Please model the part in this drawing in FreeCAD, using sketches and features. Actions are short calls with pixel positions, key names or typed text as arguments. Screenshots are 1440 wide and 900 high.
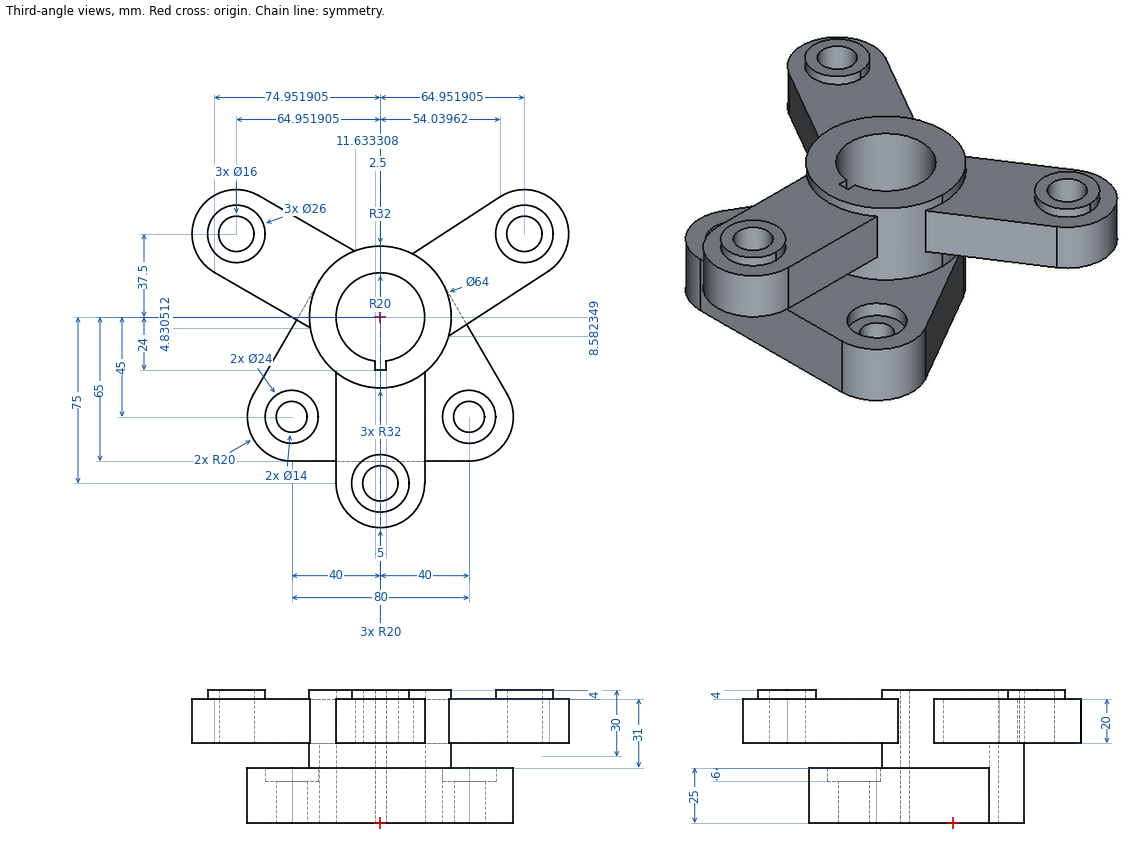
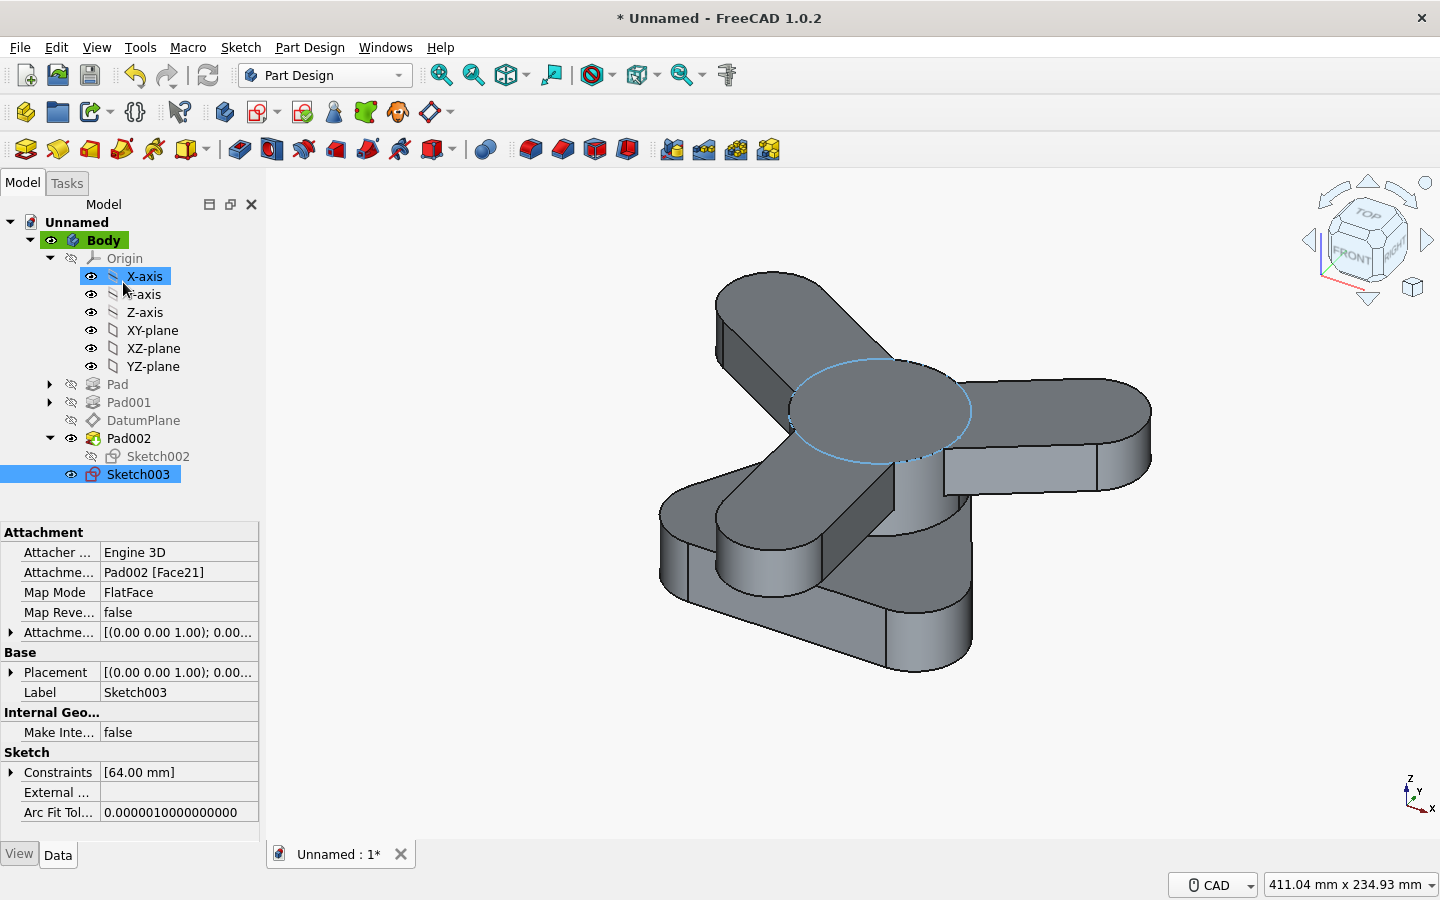
click(26, 150)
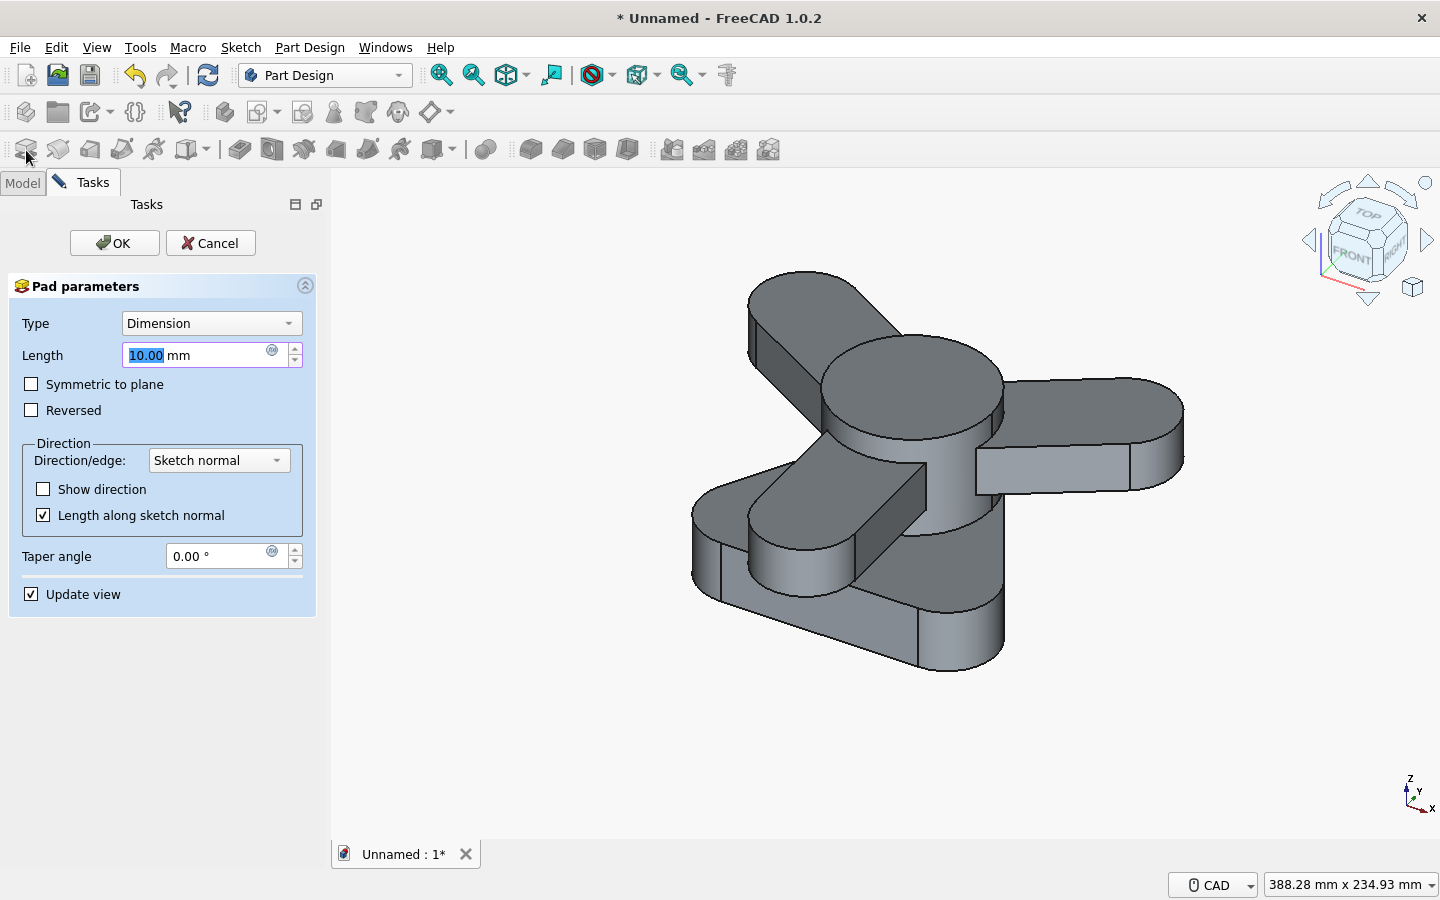
text(4)
key(Tab)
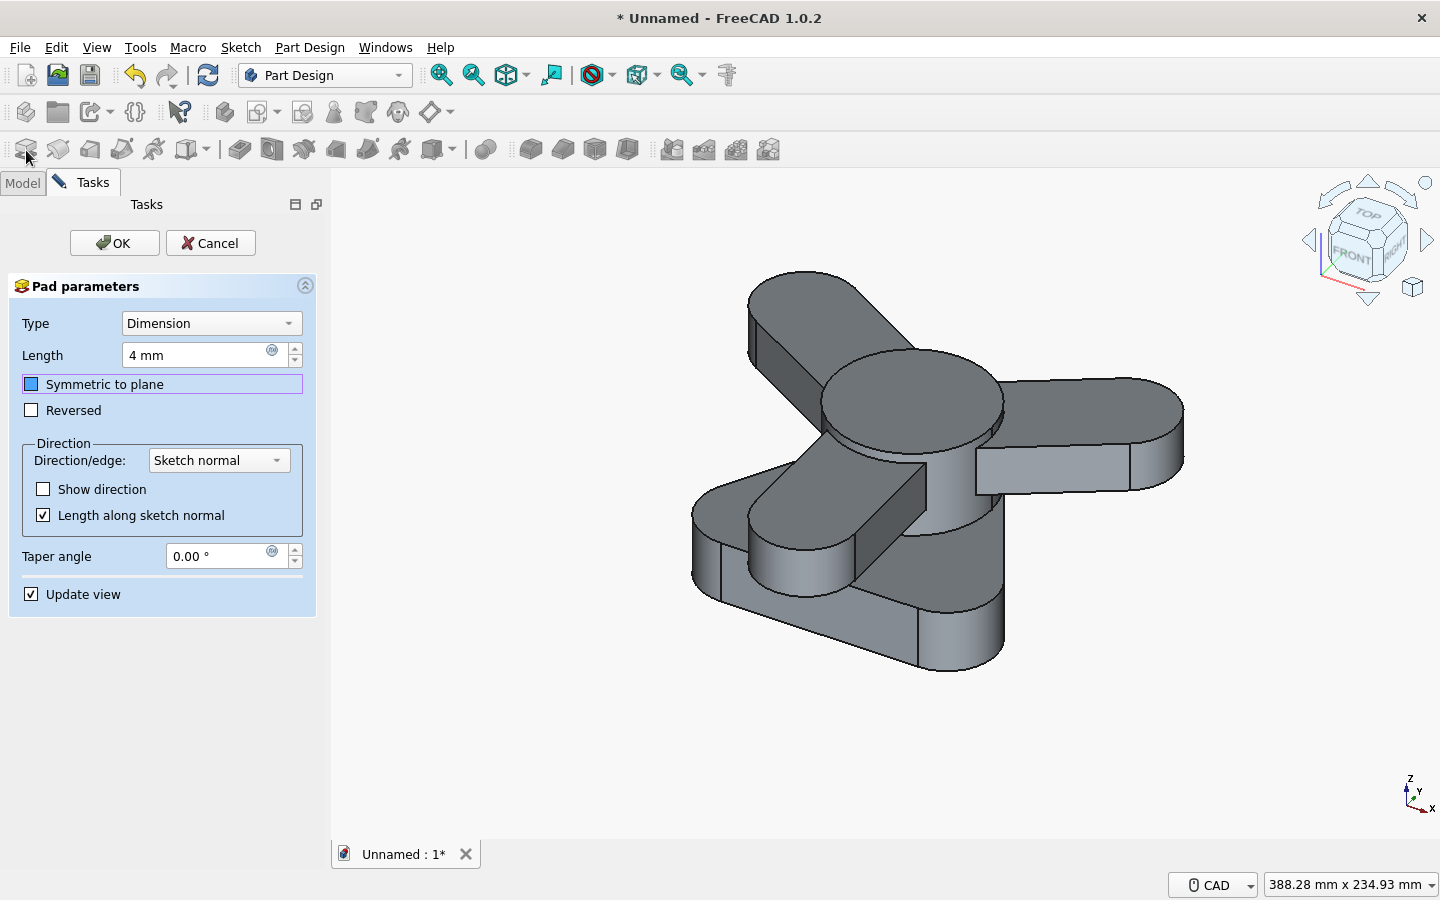
click(115, 243)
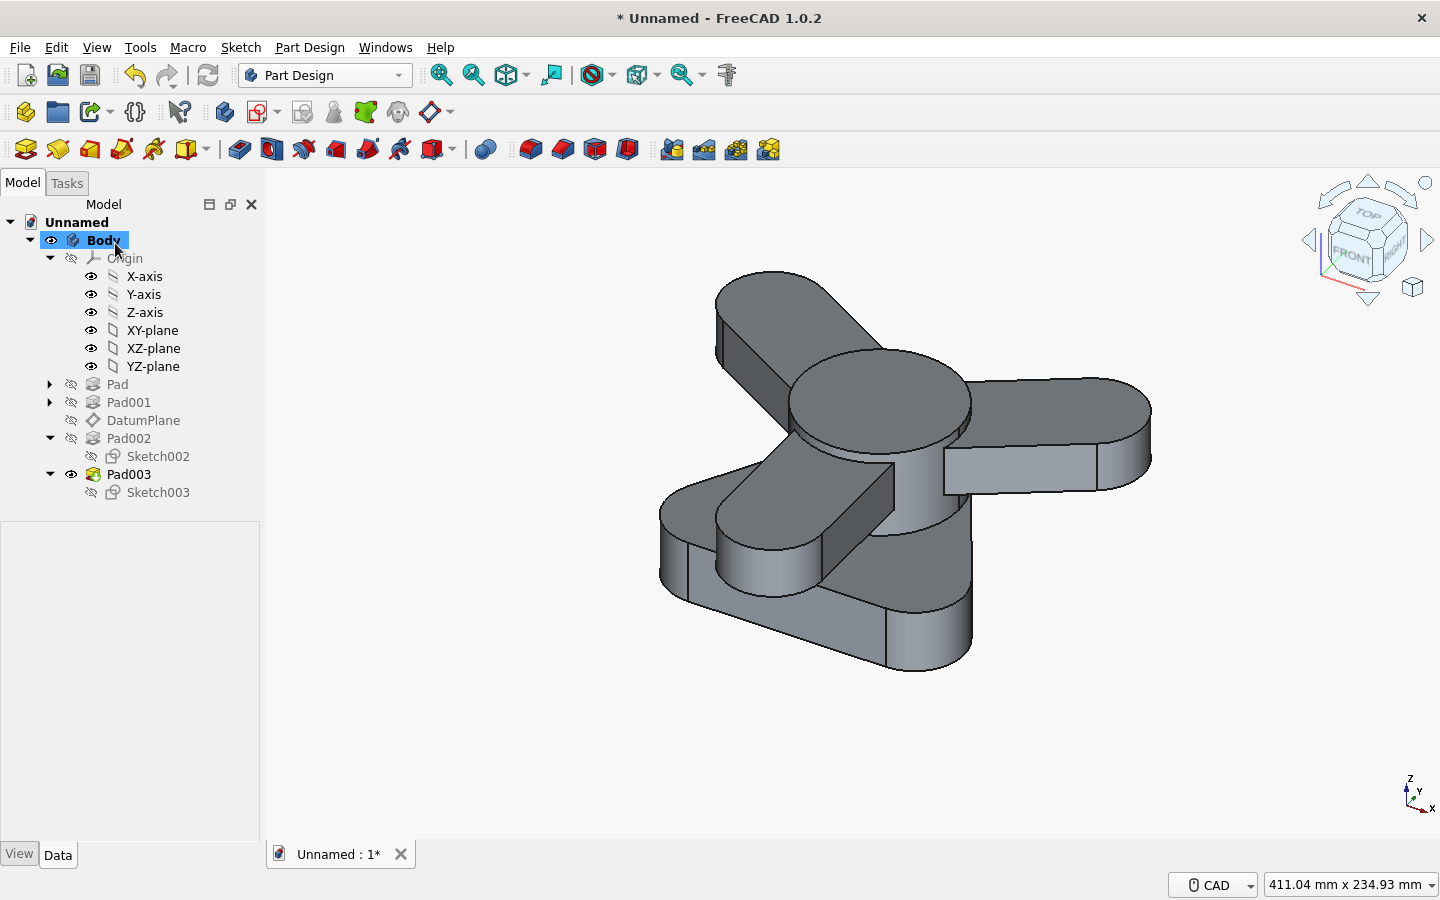
click(880, 401)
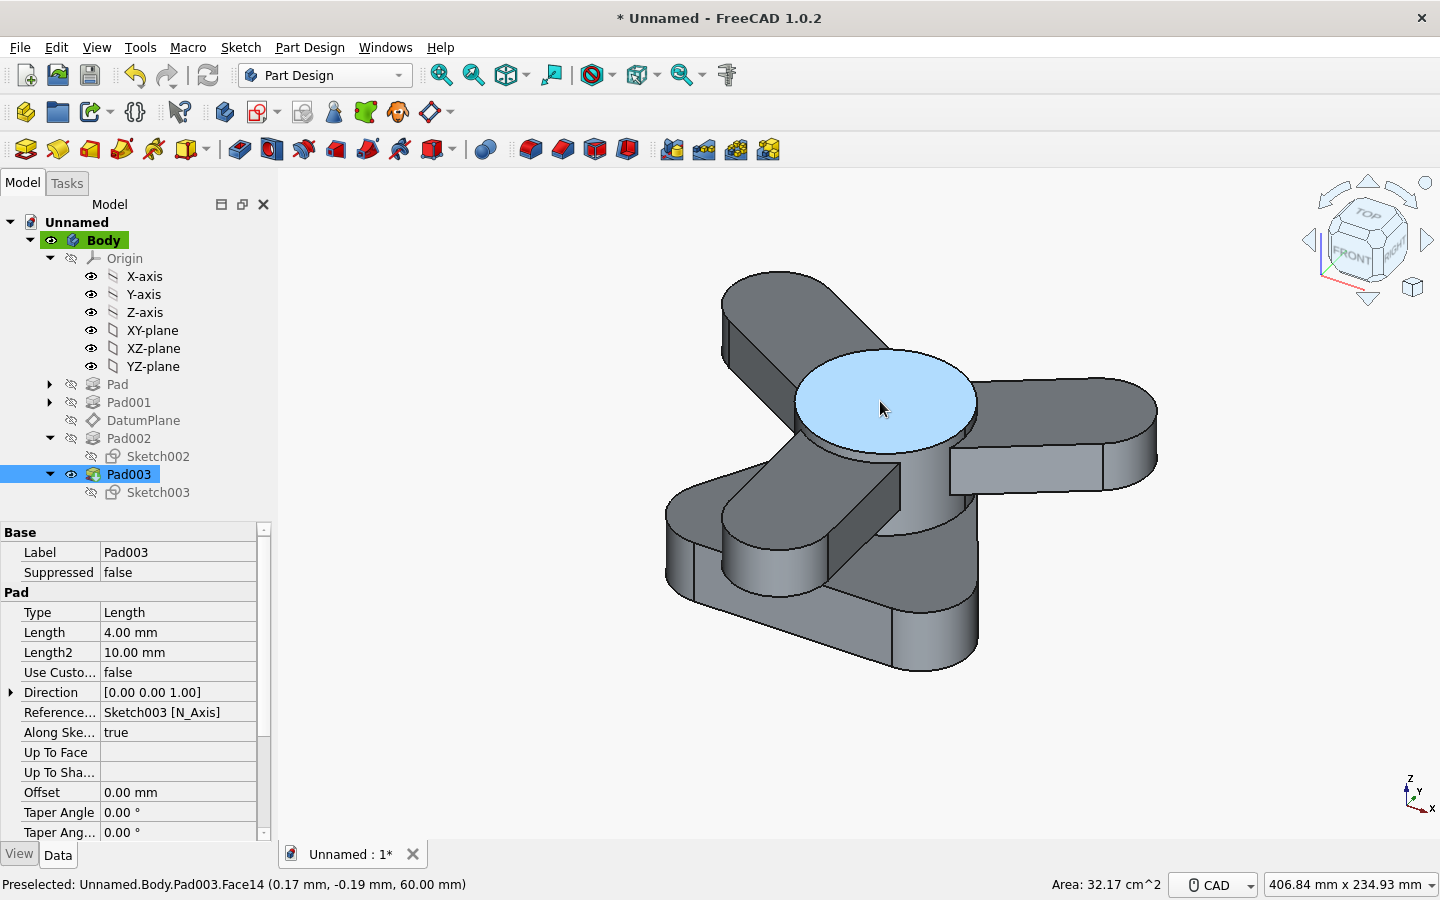
click(258, 112)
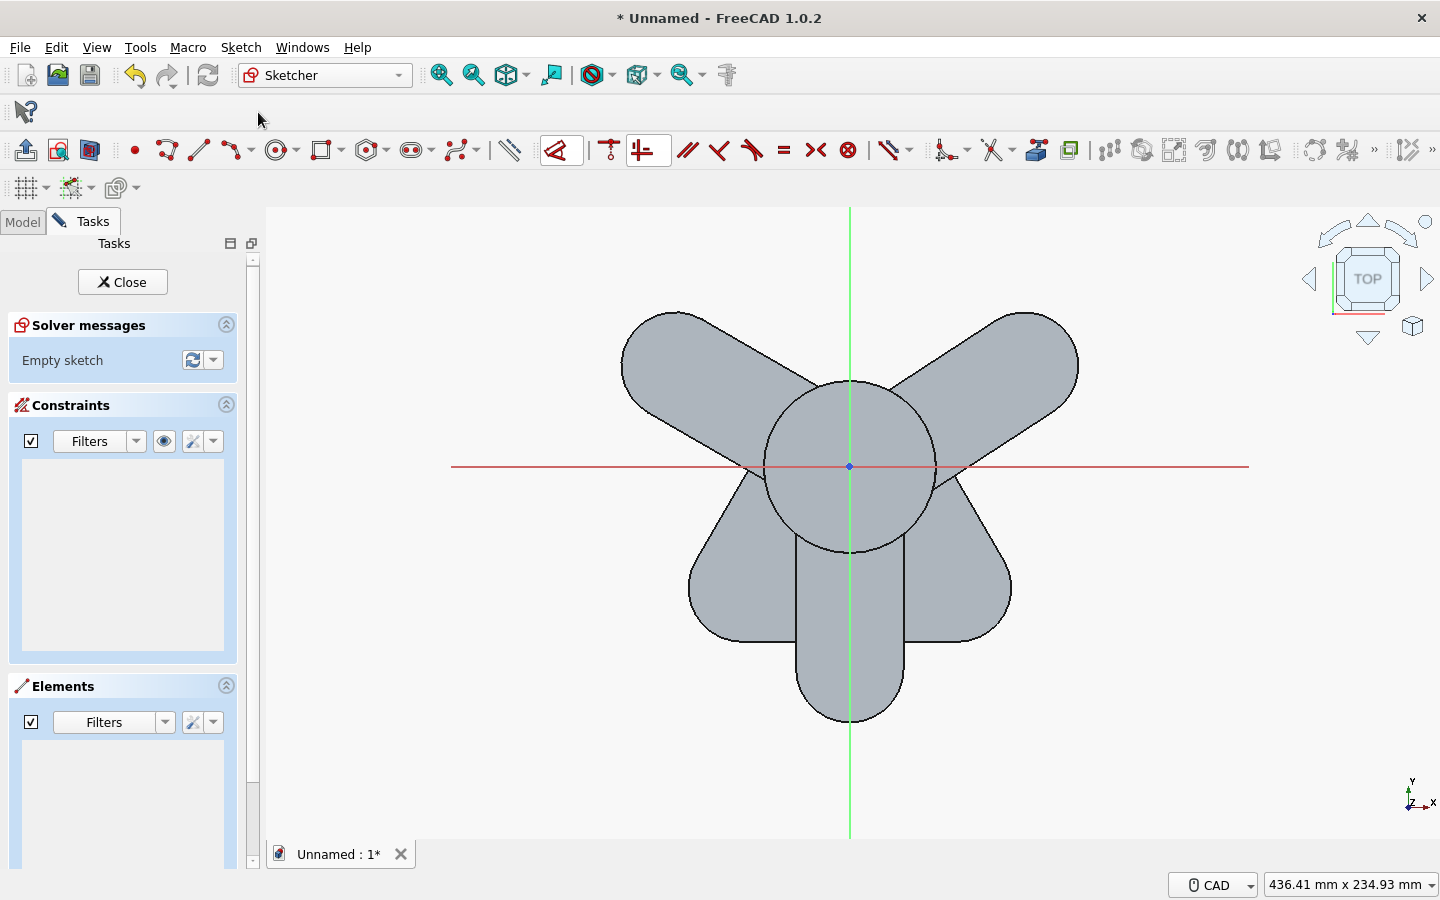
scroll(878, 451, up, 6)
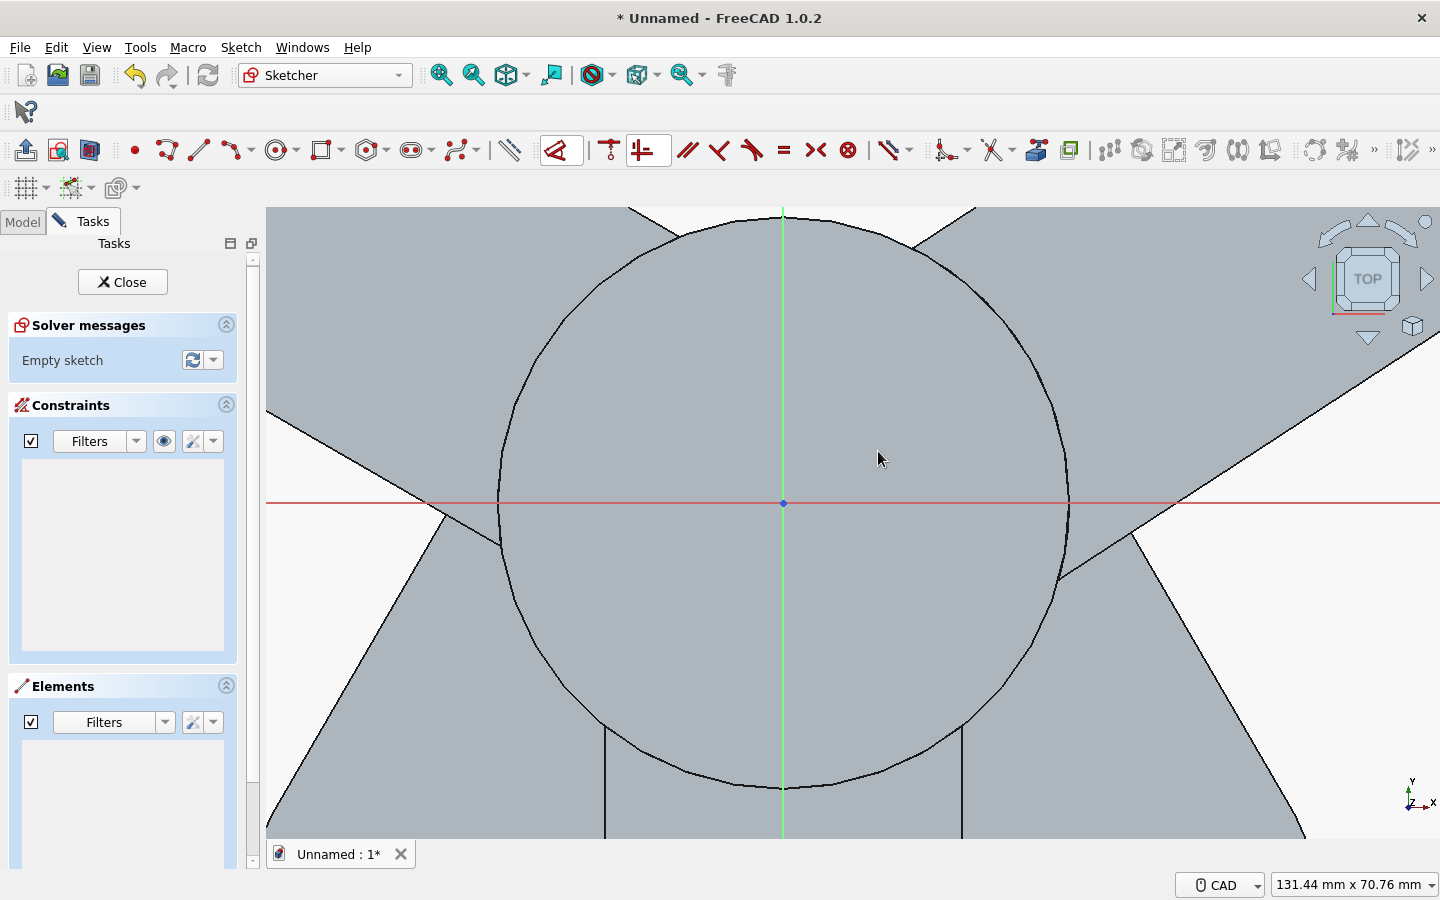
click(168, 150)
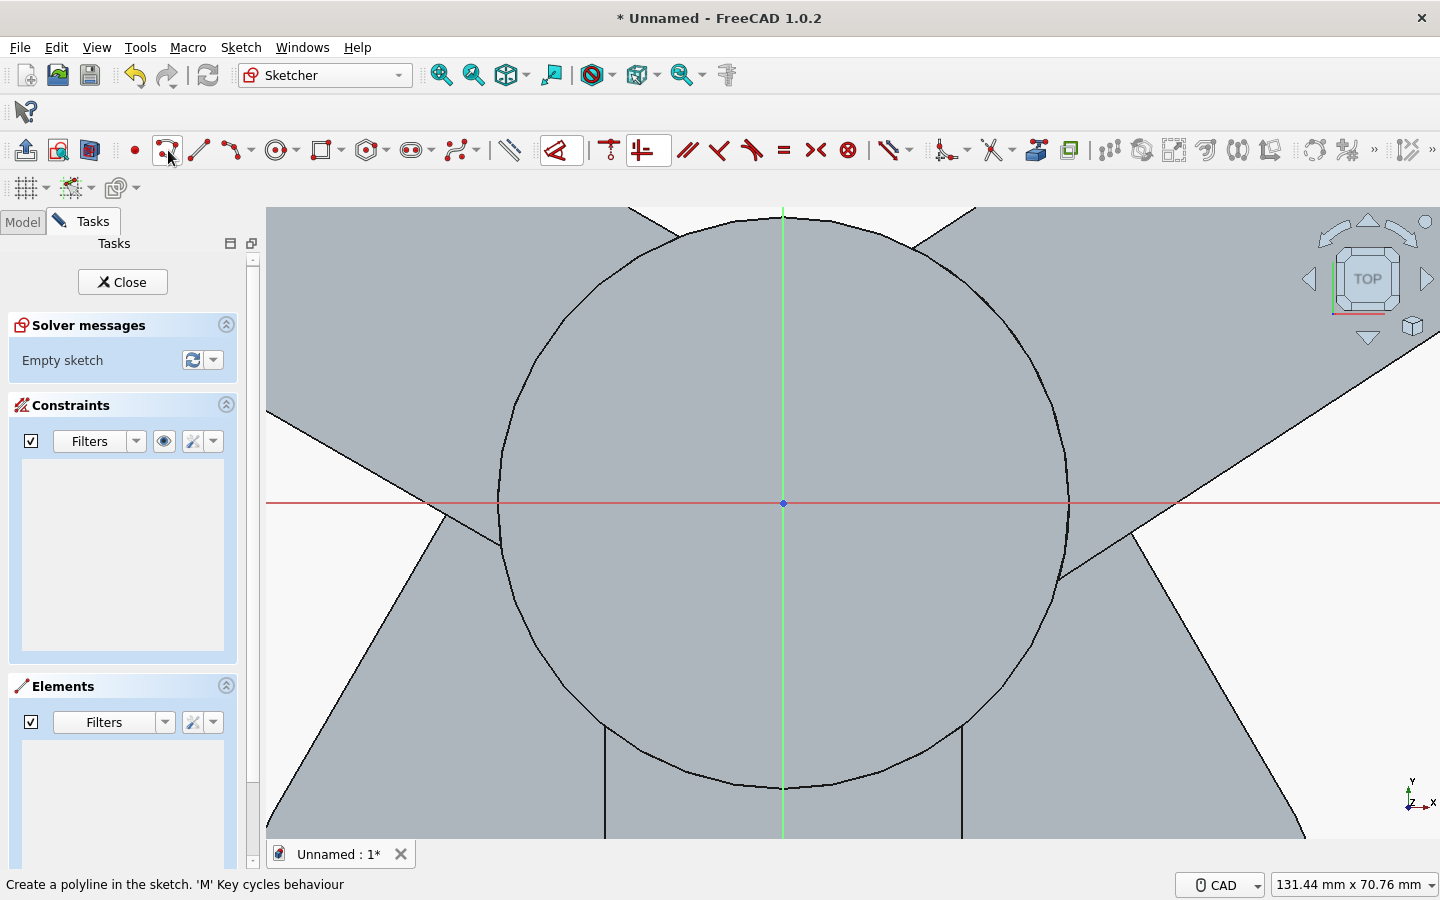
click(761, 680)
click(761, 717)
click(806, 717)
click(806, 680)
right_click(806, 680)